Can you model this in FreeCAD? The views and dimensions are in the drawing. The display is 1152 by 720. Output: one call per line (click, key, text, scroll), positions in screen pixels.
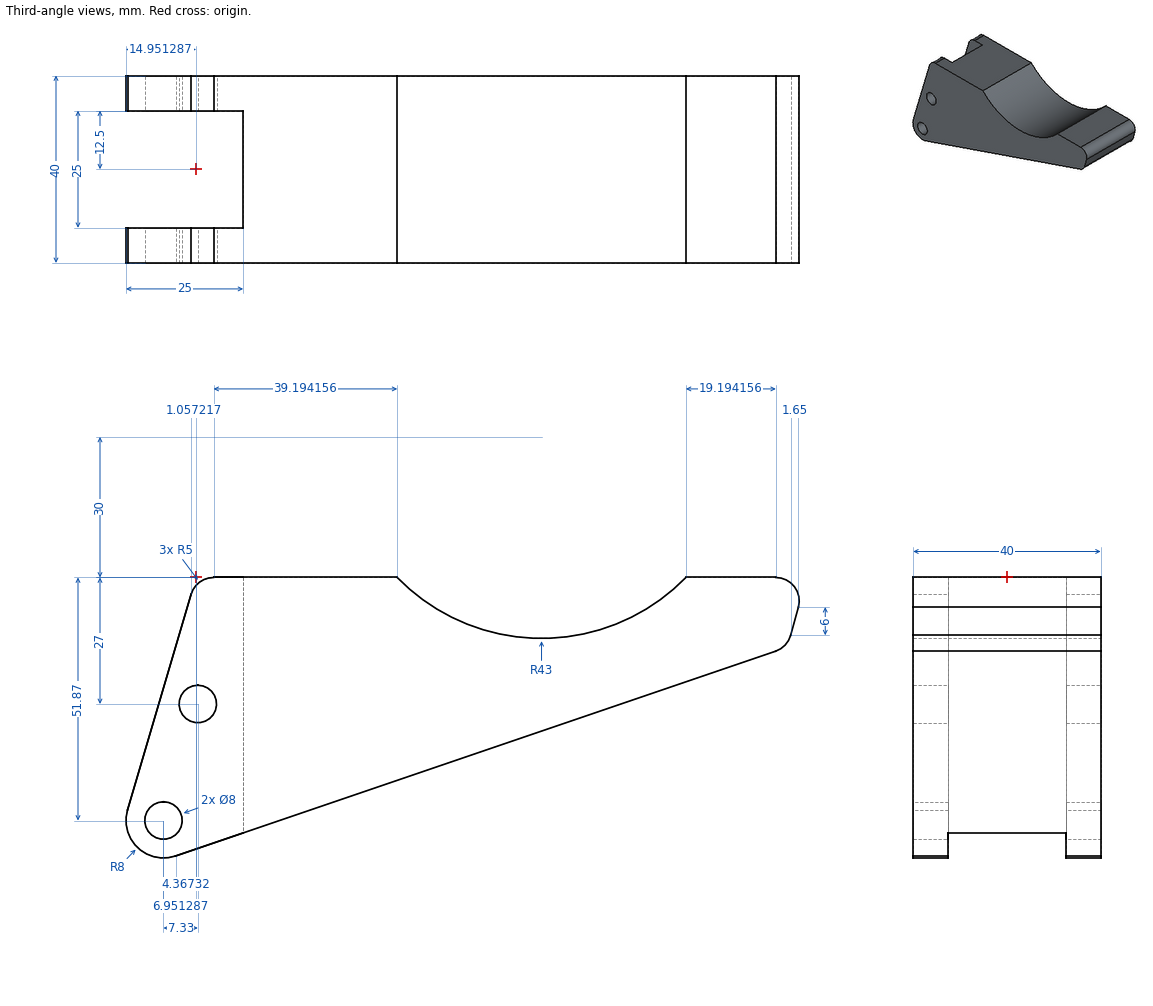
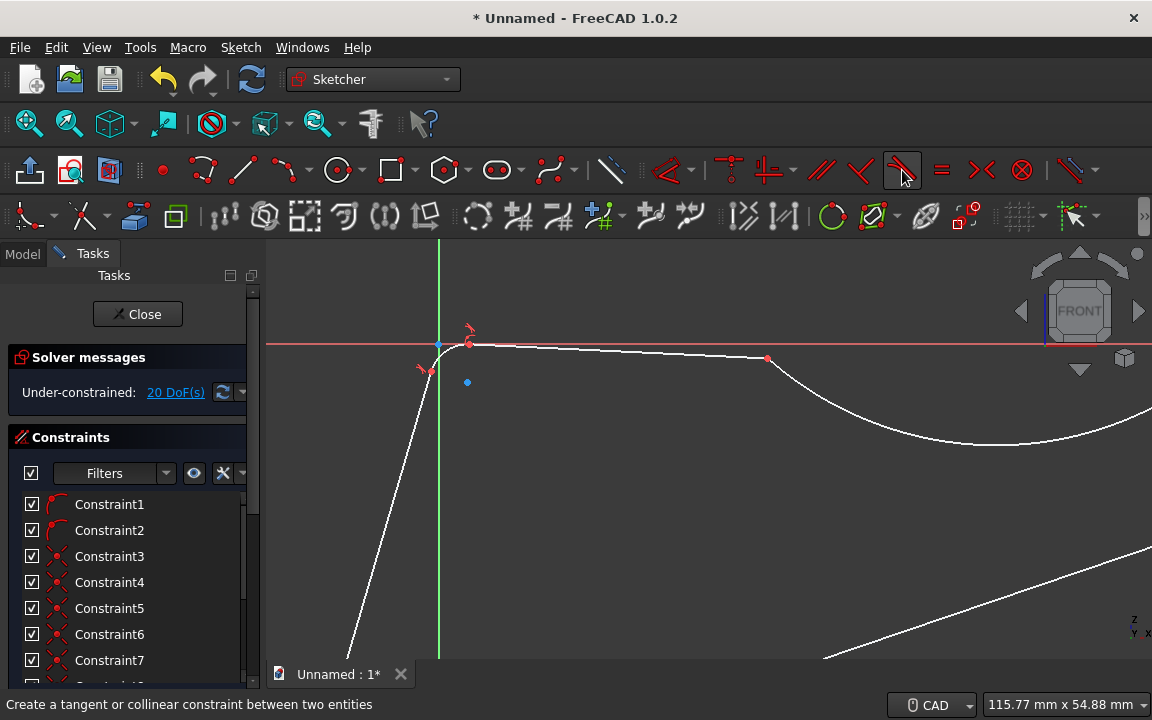
scroll(449, 349, down, 4)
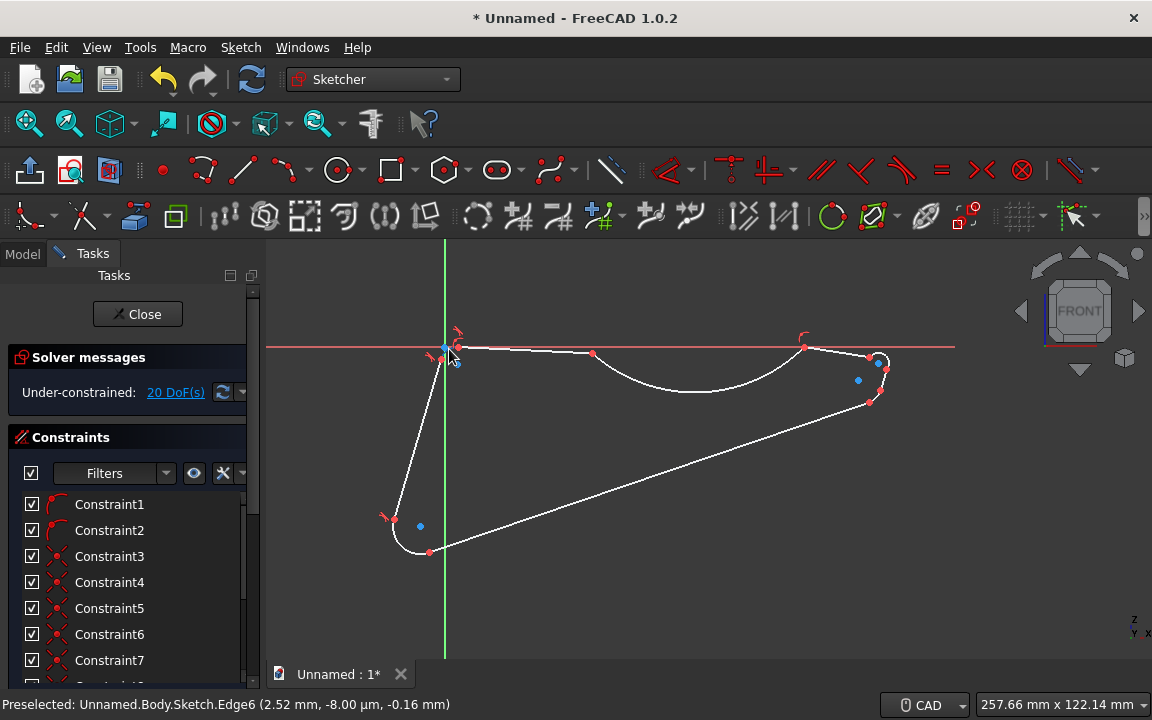
scroll(850, 354, up, 4)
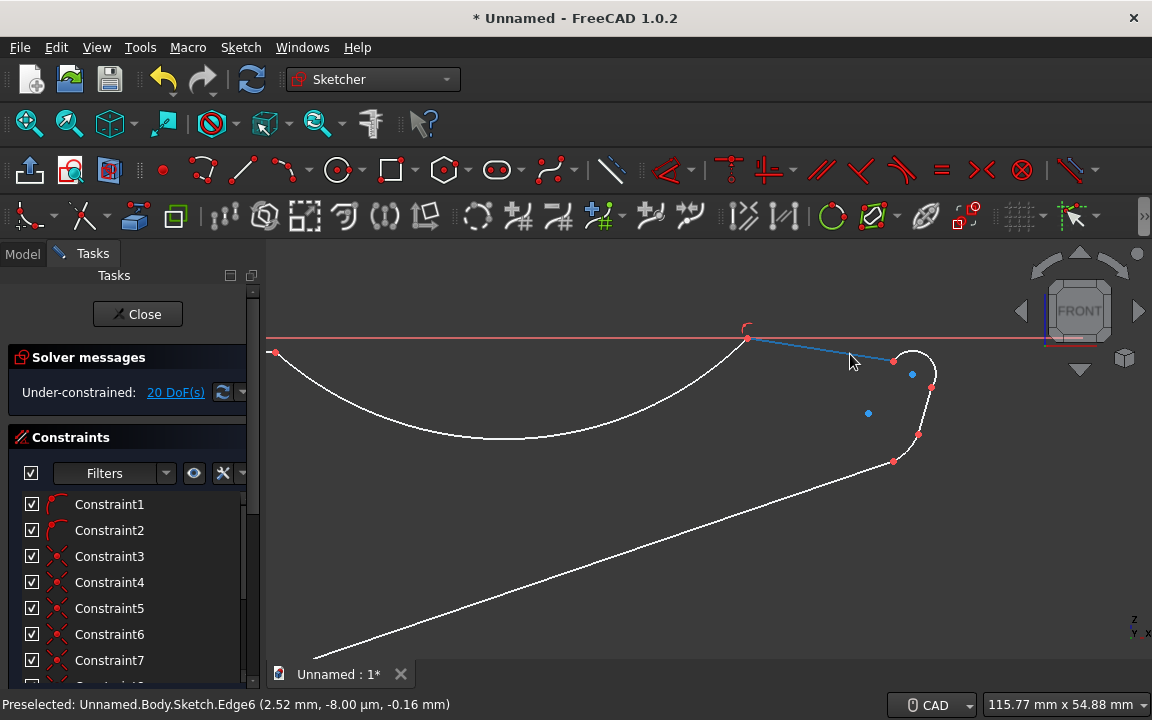
click(850, 354)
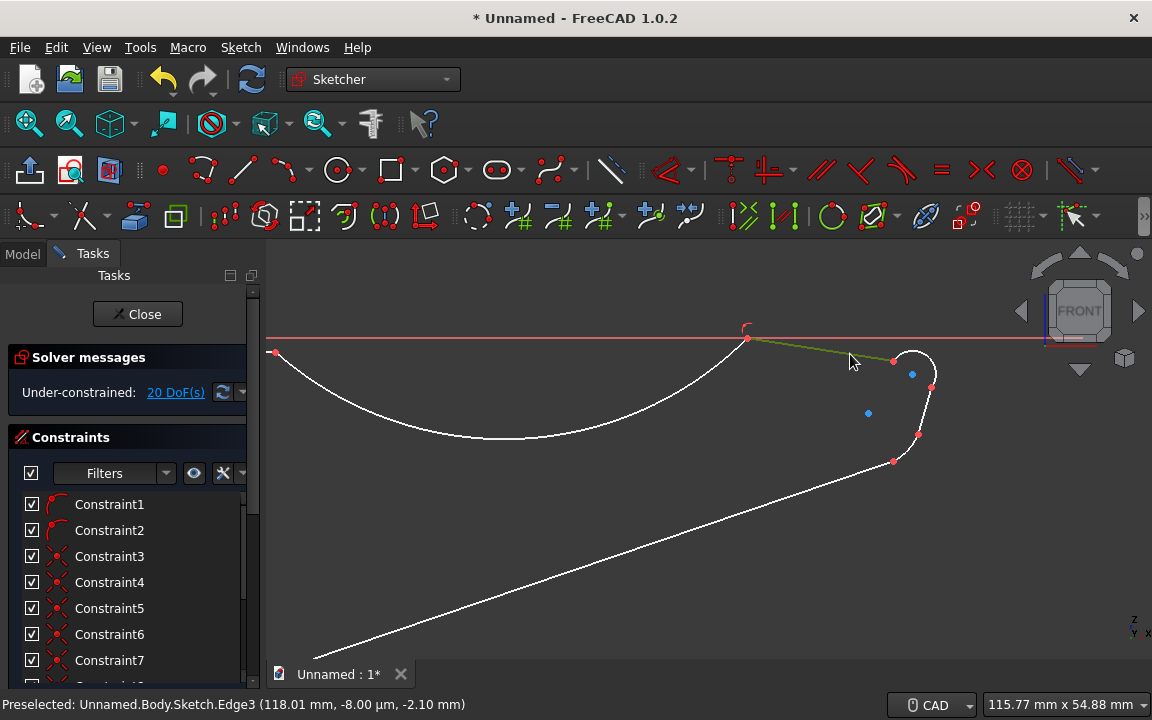
click(935, 367)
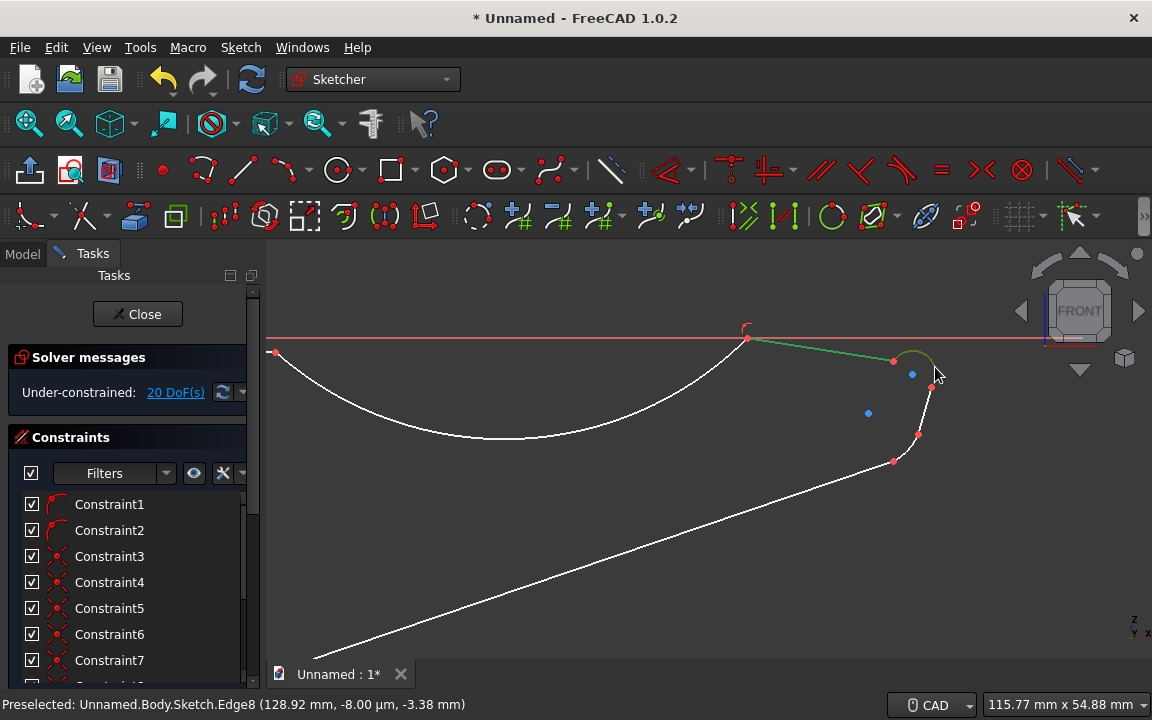
click(902, 170)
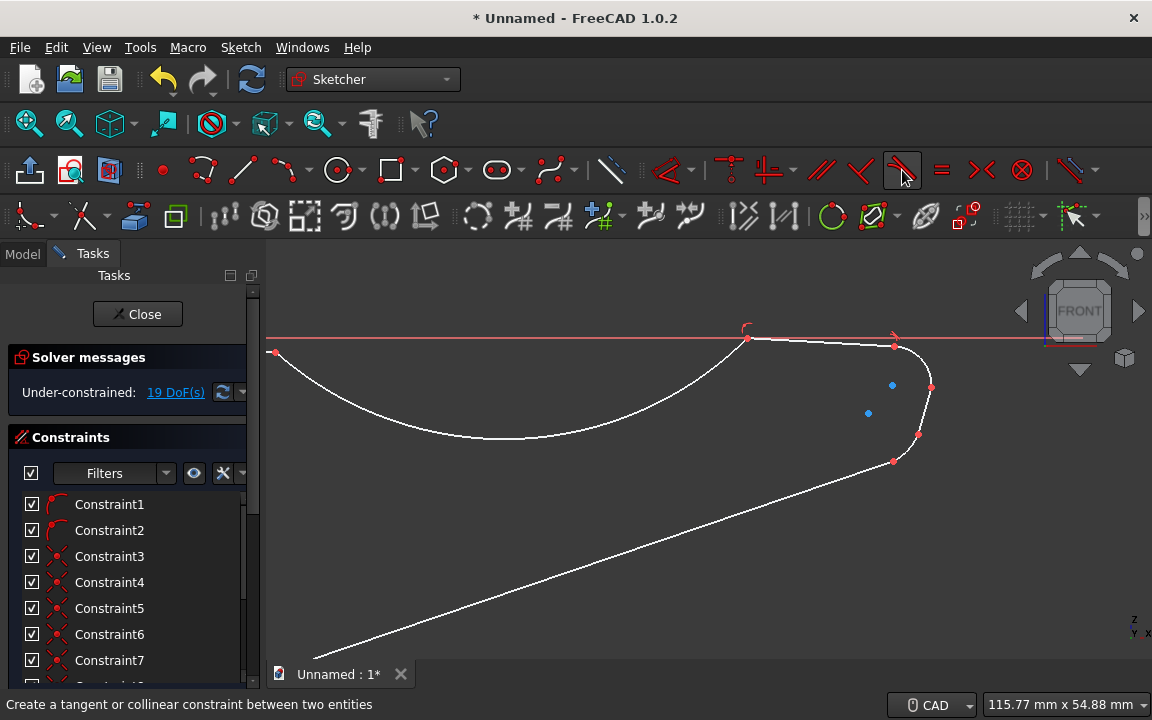
click(927, 402)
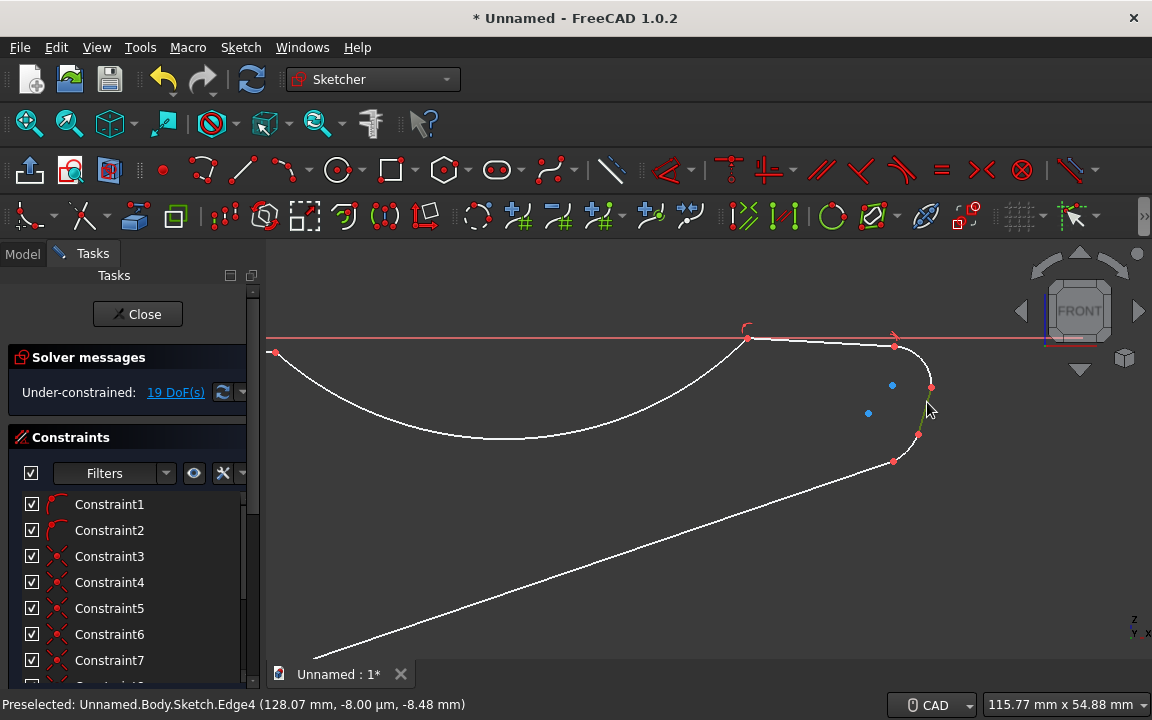
click(928, 370)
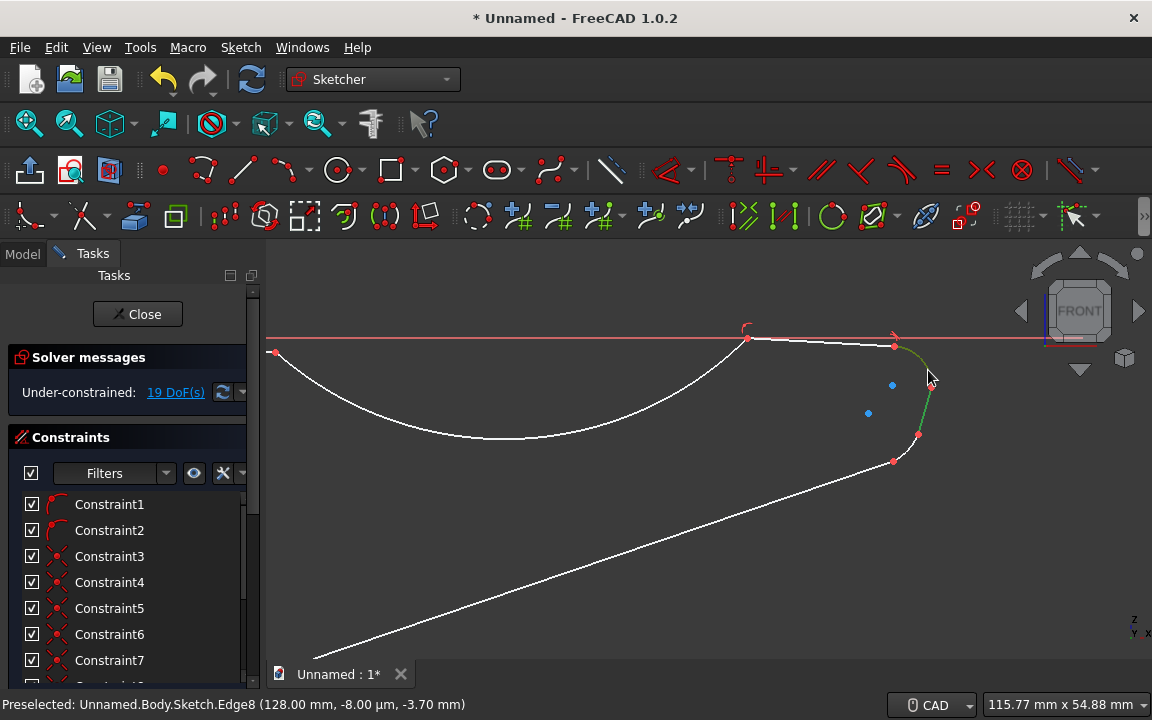
click(902, 170)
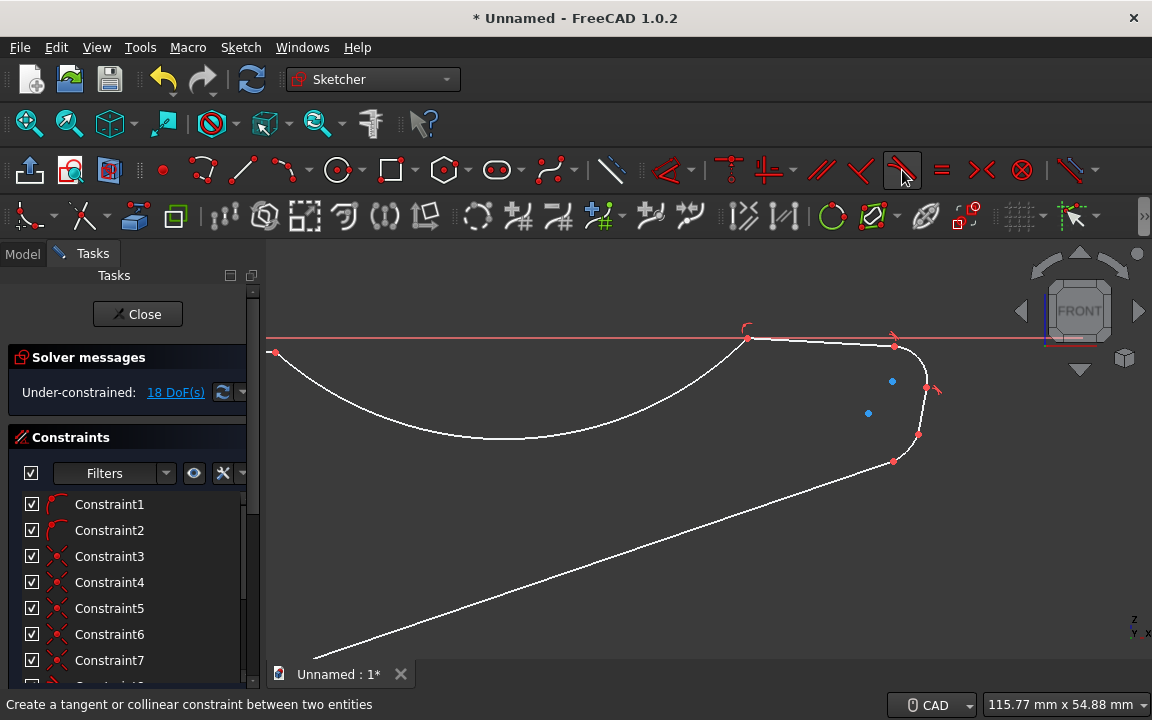
click(924, 402)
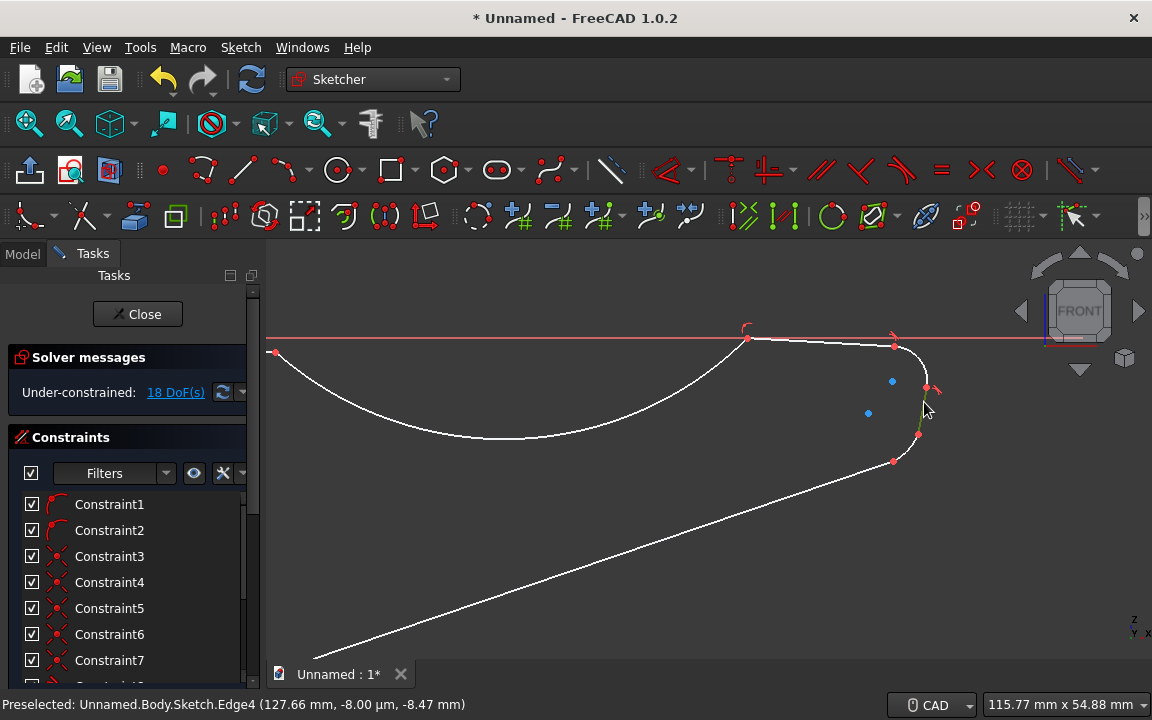
scroll(903, 455, up, 2)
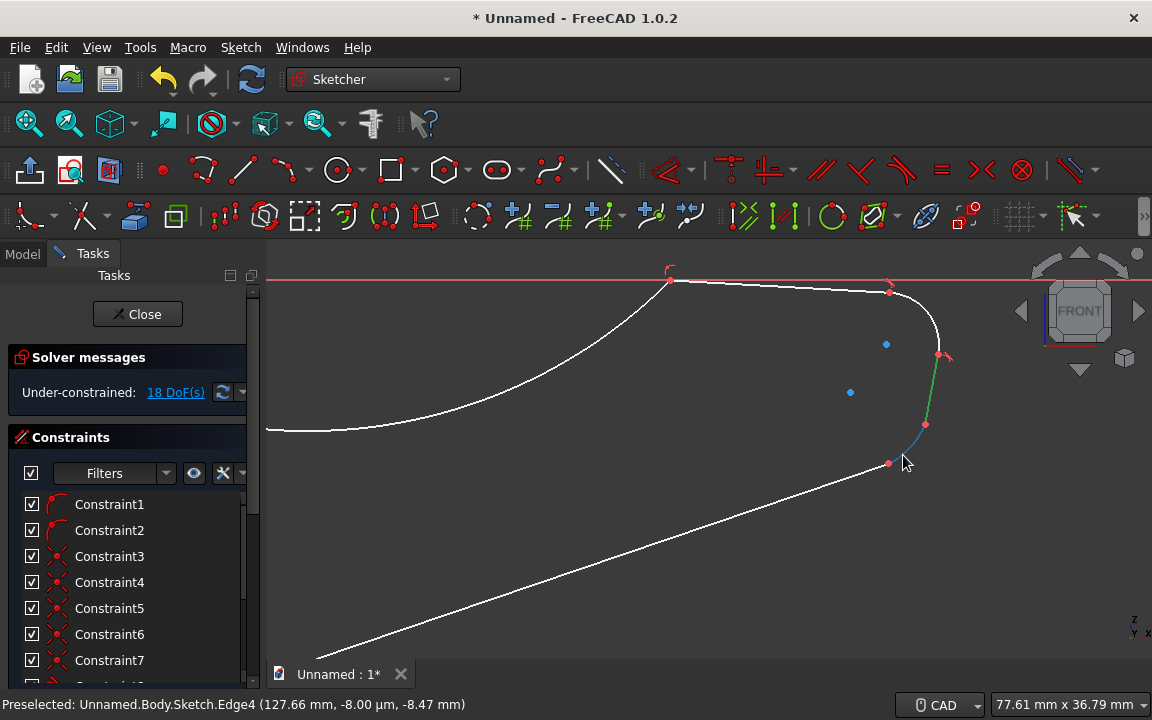
click(902, 455)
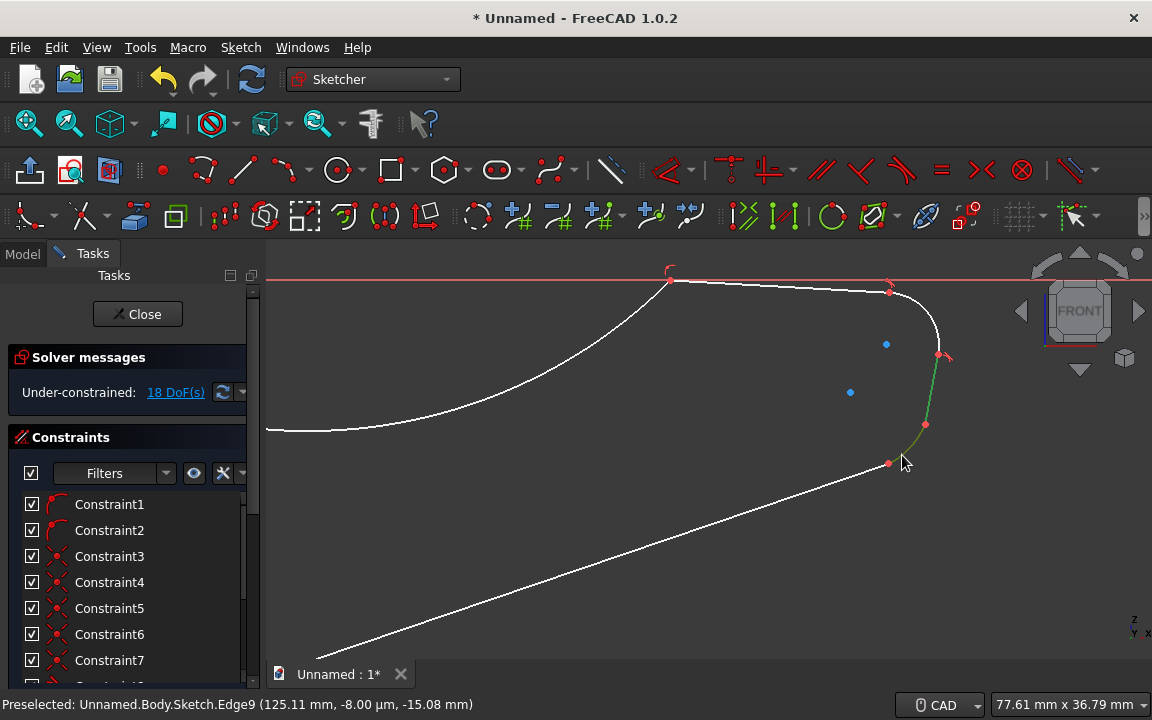
click(902, 170)